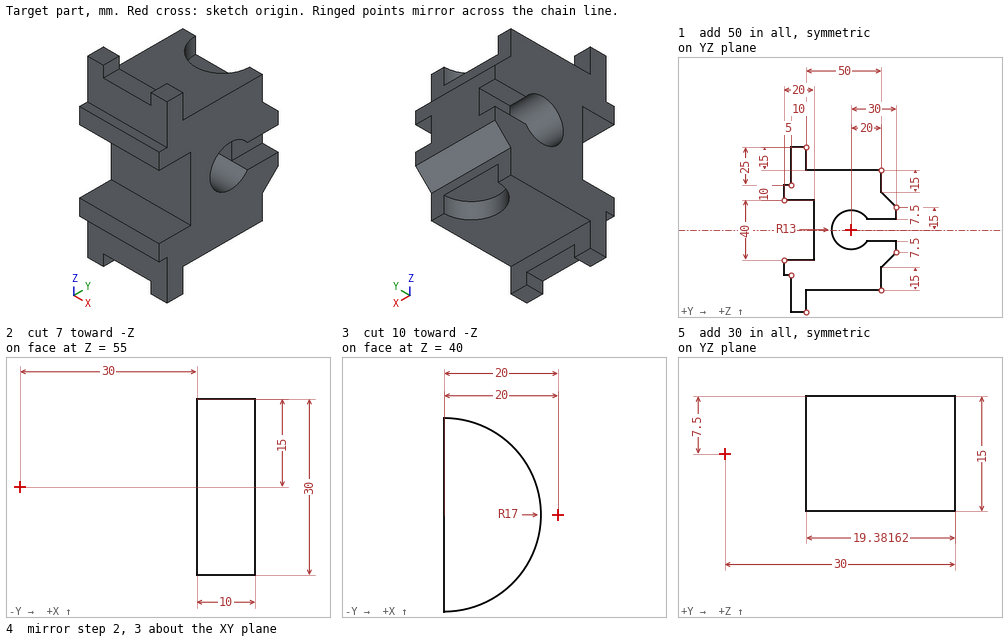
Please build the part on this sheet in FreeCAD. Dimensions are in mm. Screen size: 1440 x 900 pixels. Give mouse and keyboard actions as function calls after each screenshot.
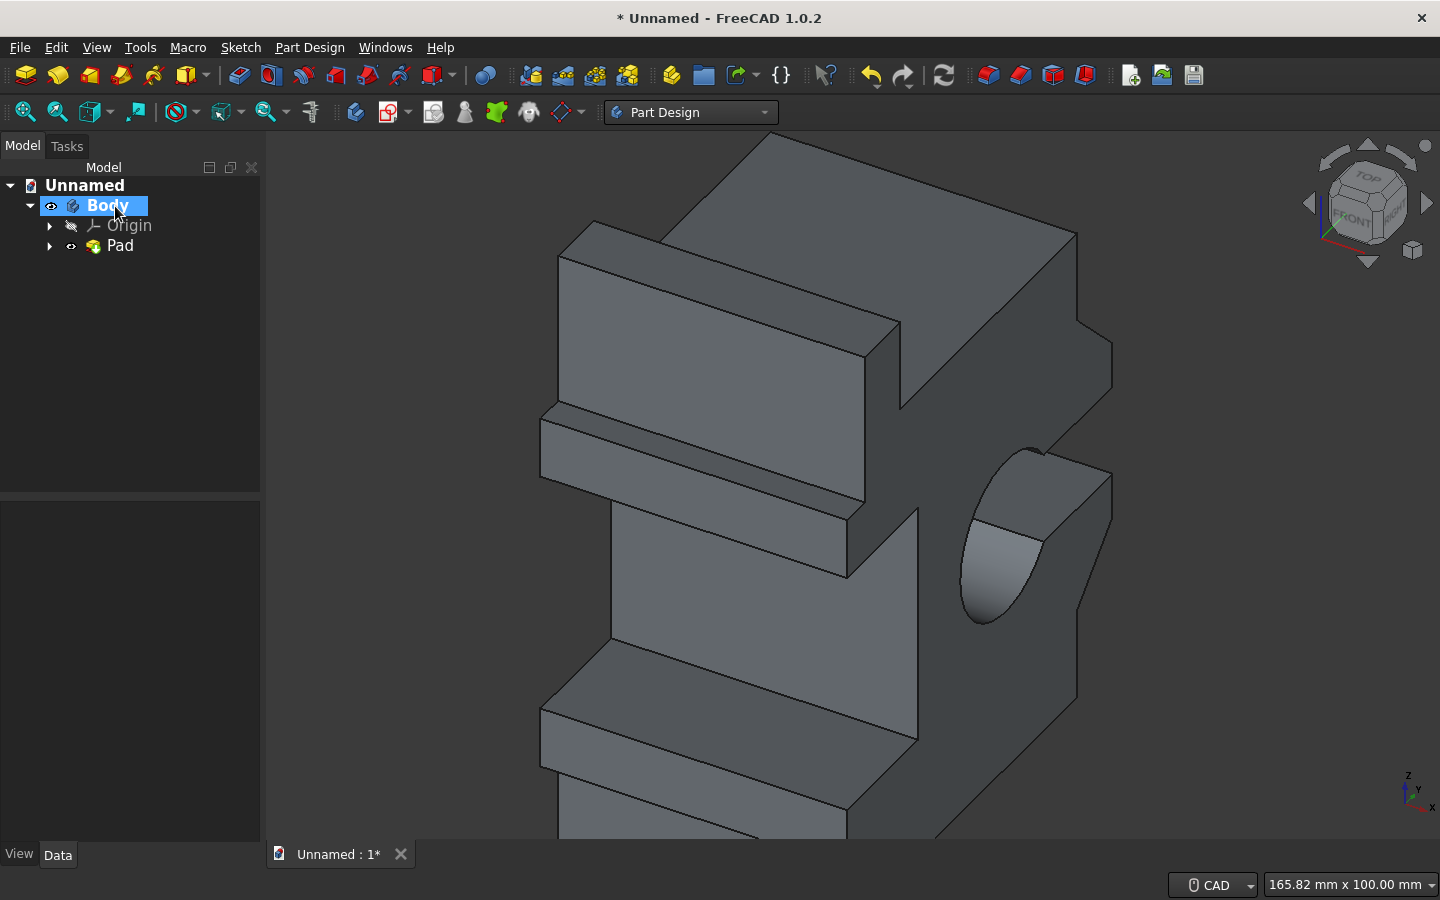
click(26, 112)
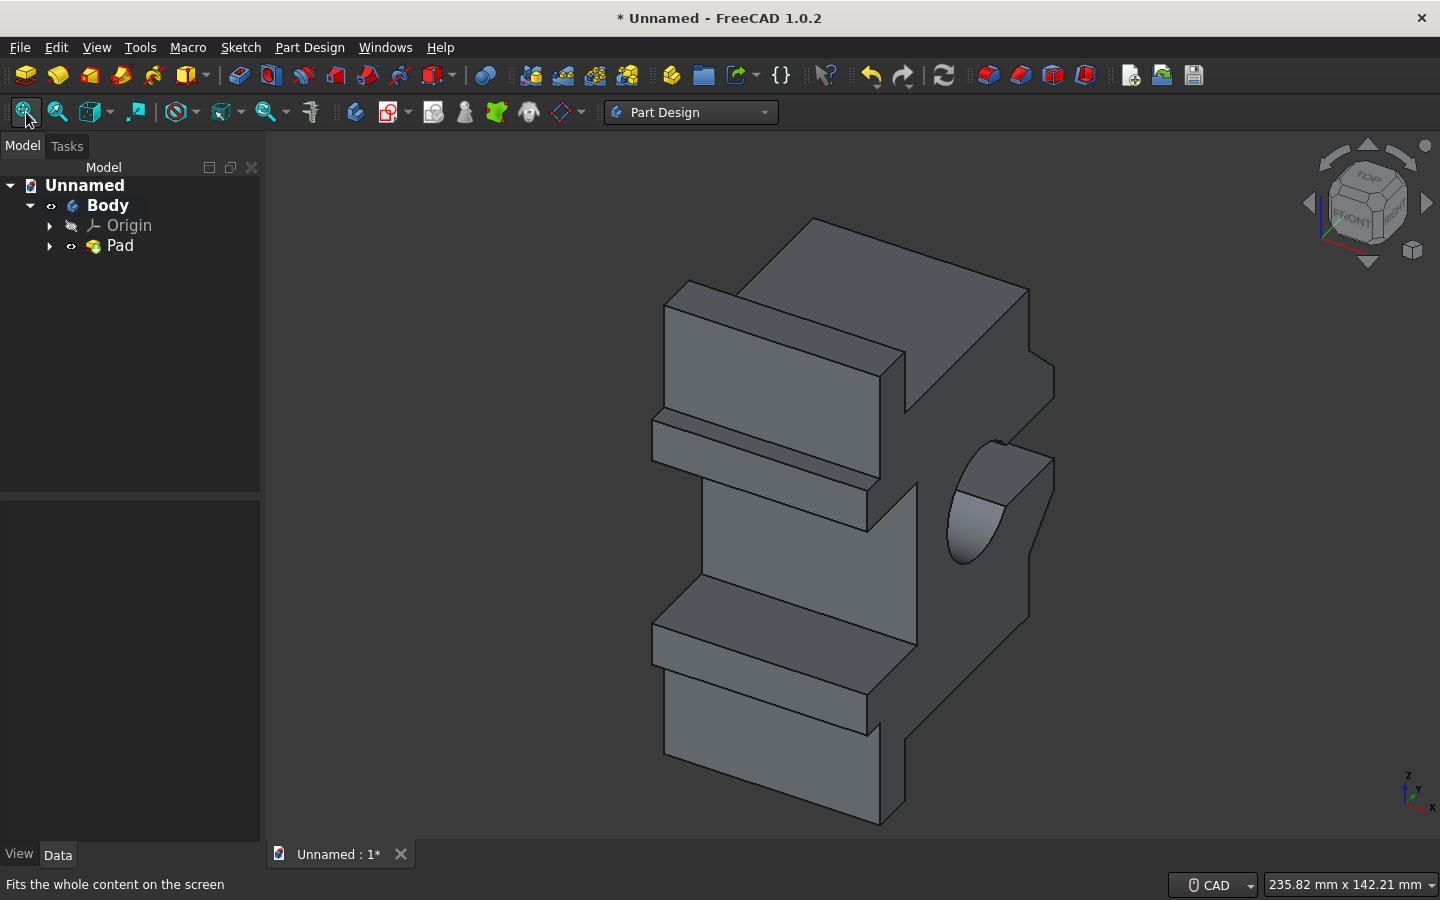
click(754, 318)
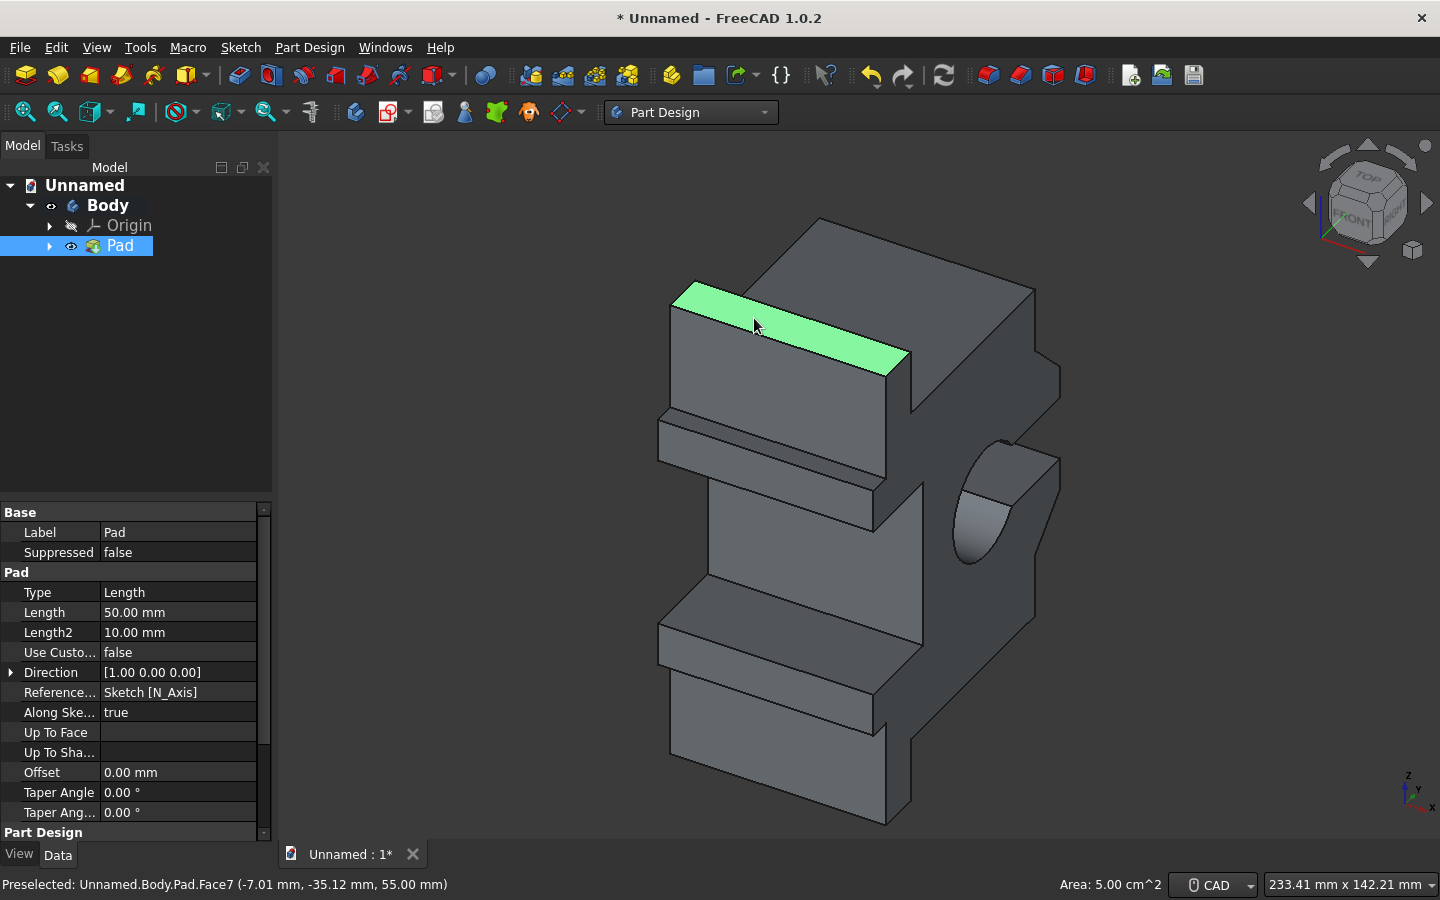
click(388, 112)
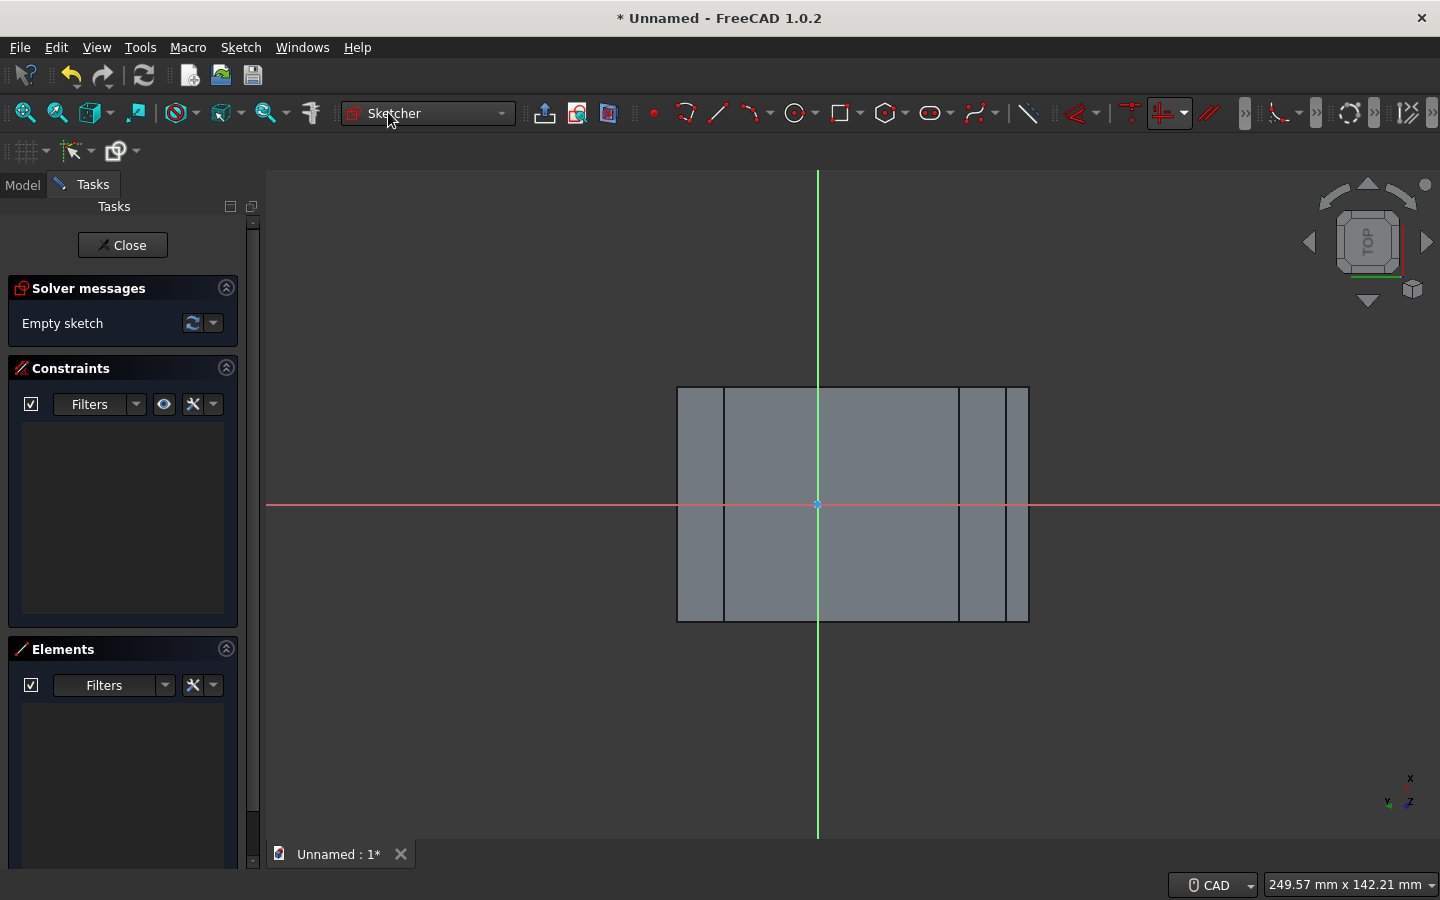
scroll(967, 504, up, 6)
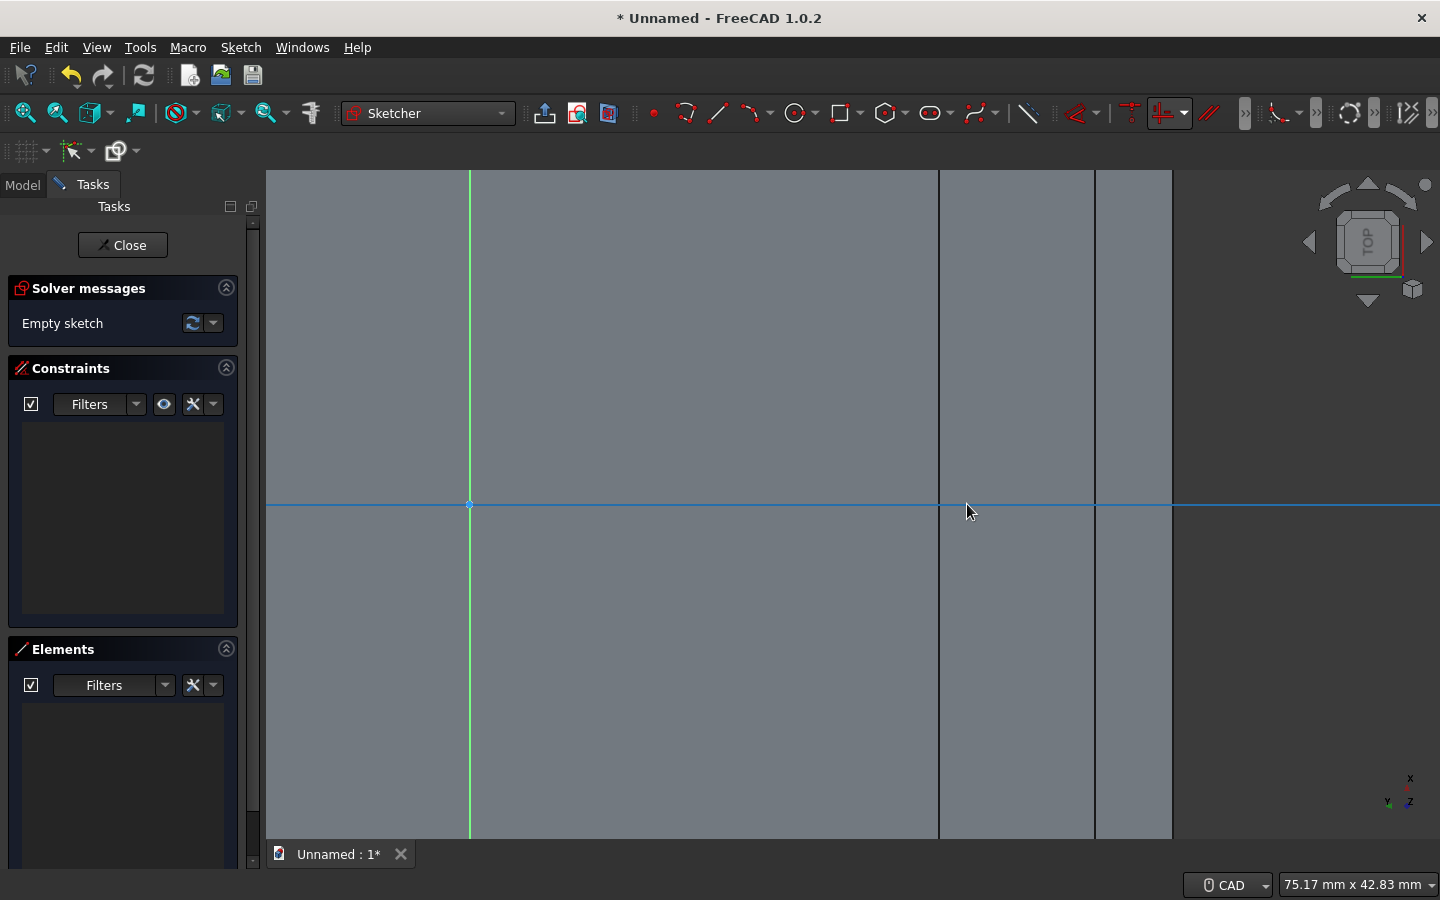
click(840, 114)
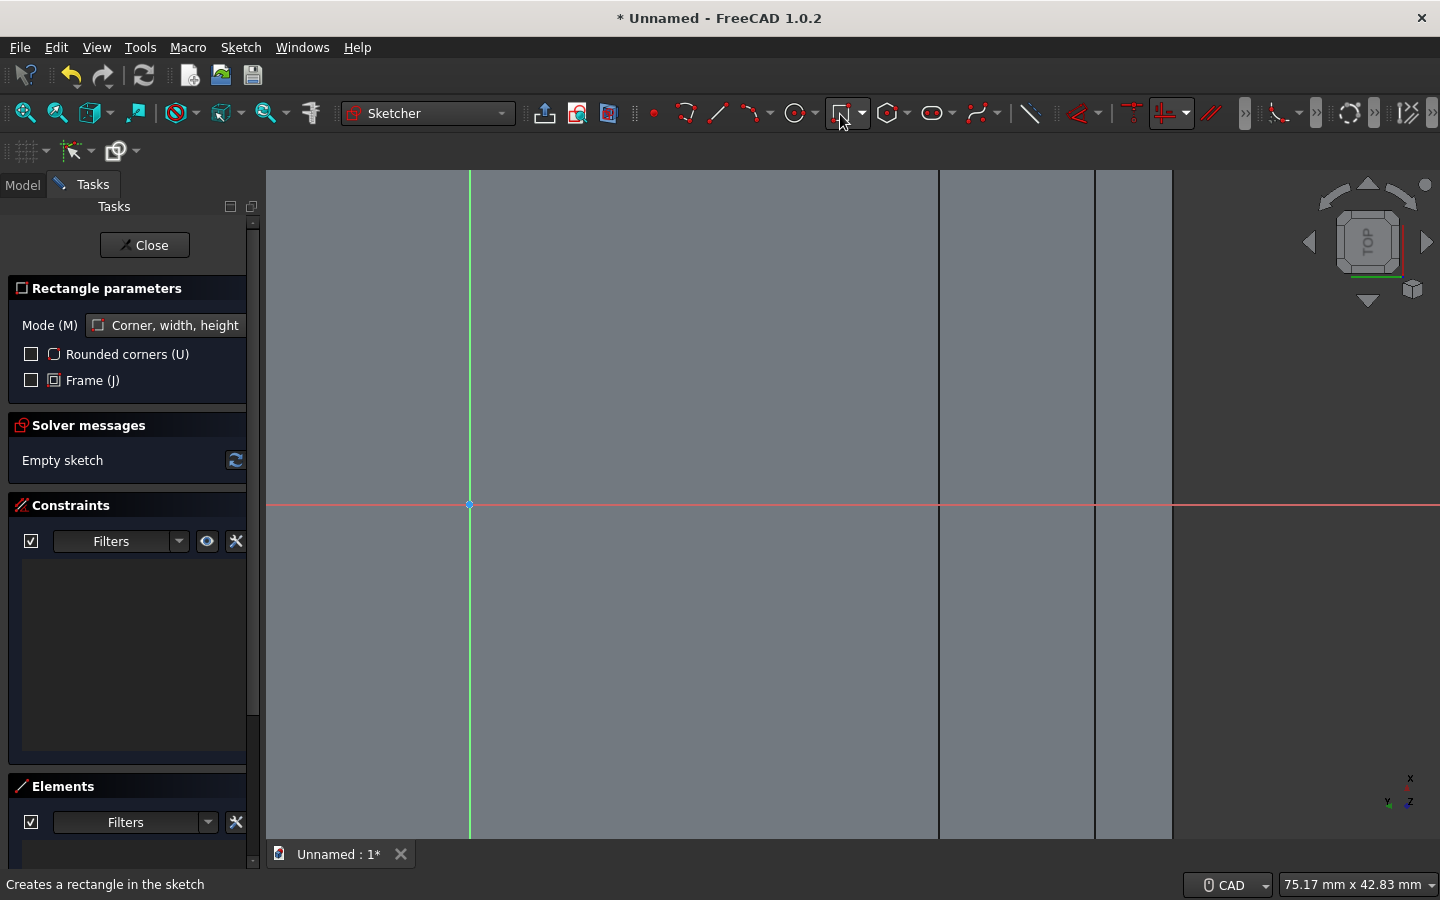
click(939, 270)
move(1095, 739)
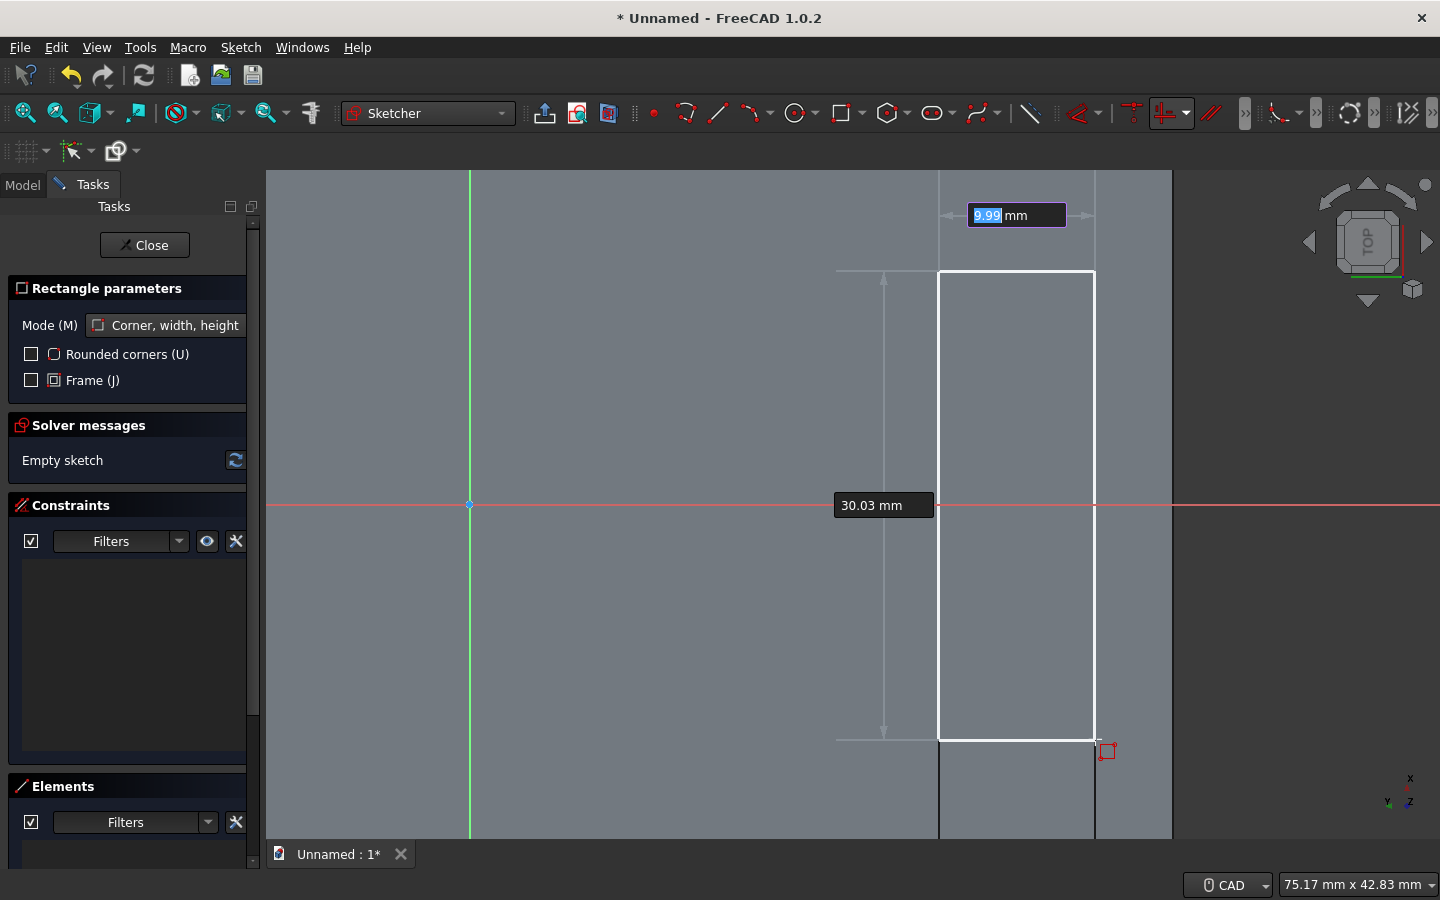
text(10)
key(Tab)
text(30)
key(Return)
key(Escape)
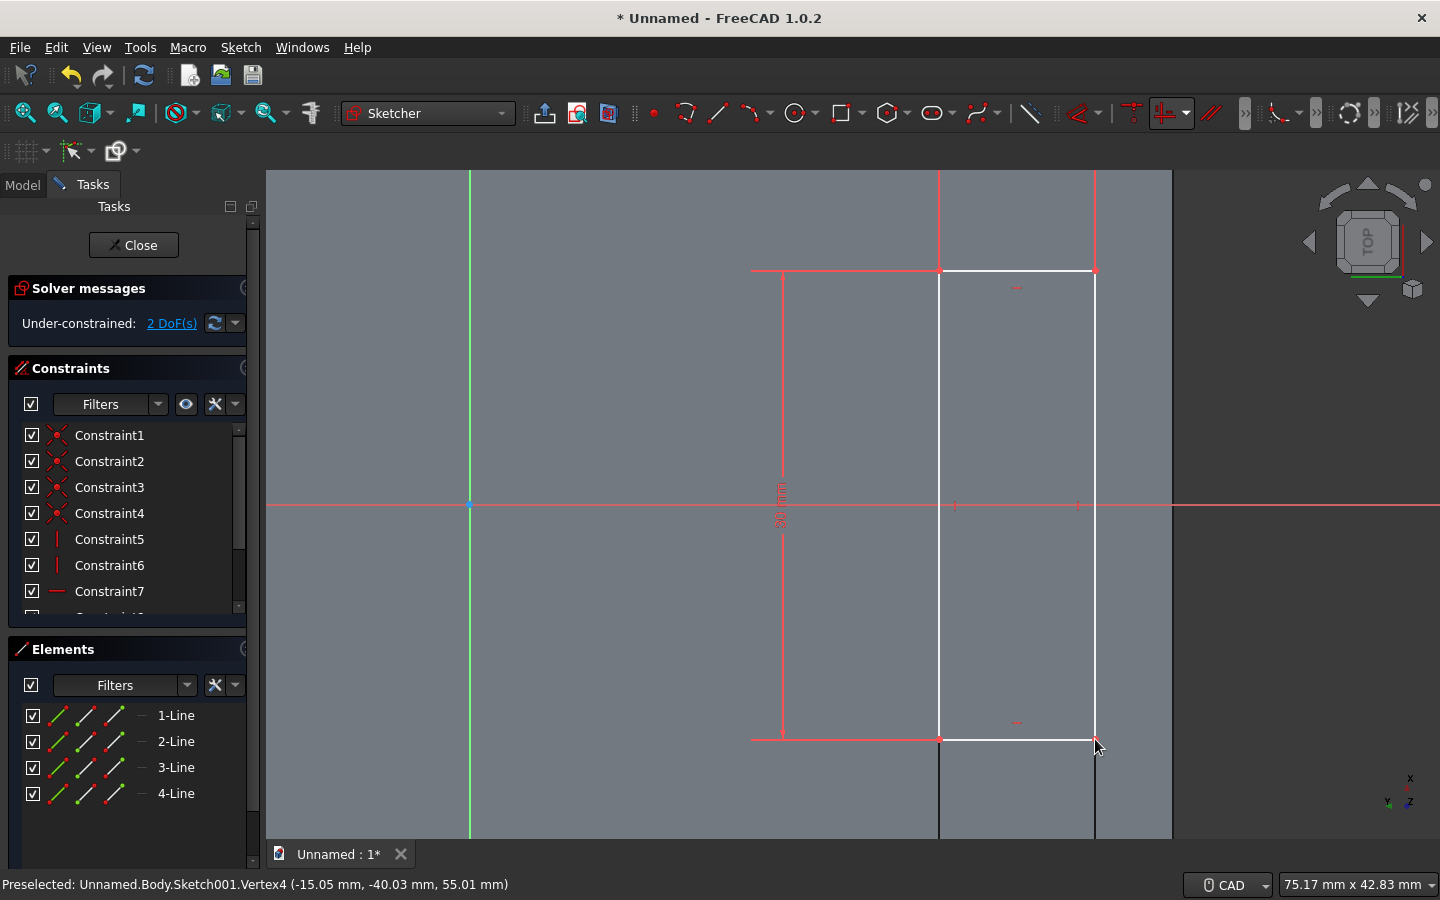
click(1078, 114)